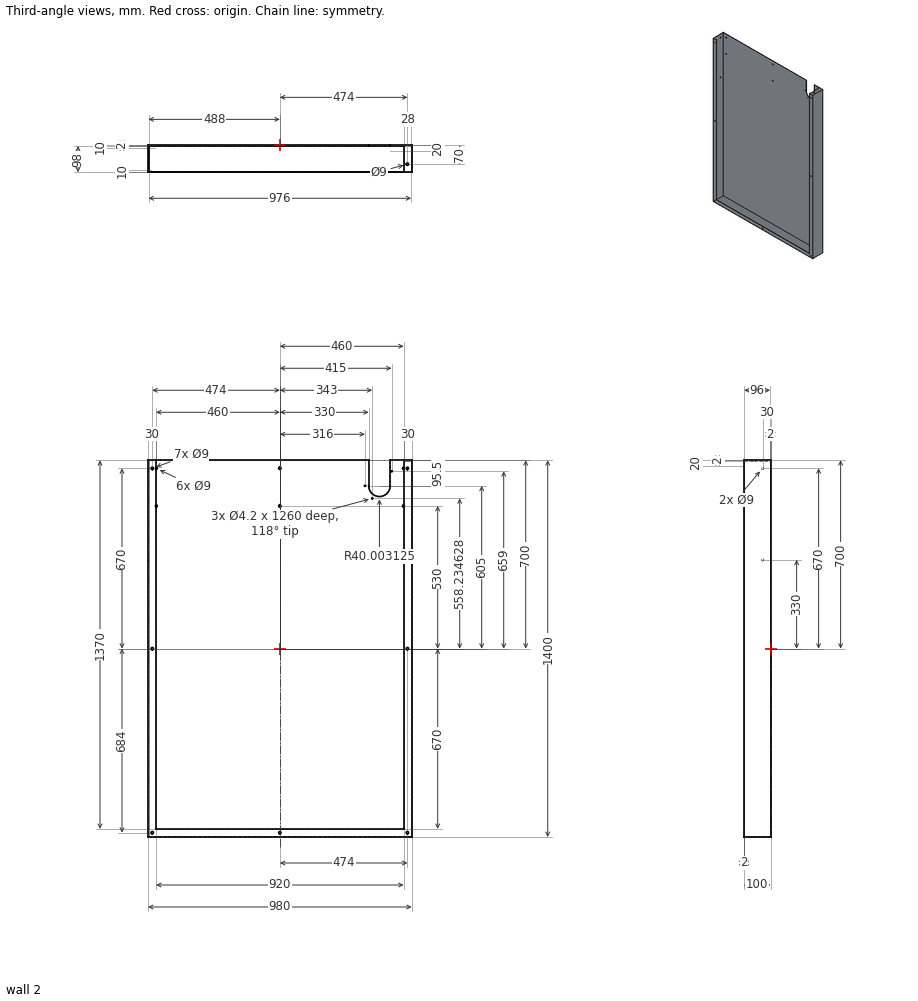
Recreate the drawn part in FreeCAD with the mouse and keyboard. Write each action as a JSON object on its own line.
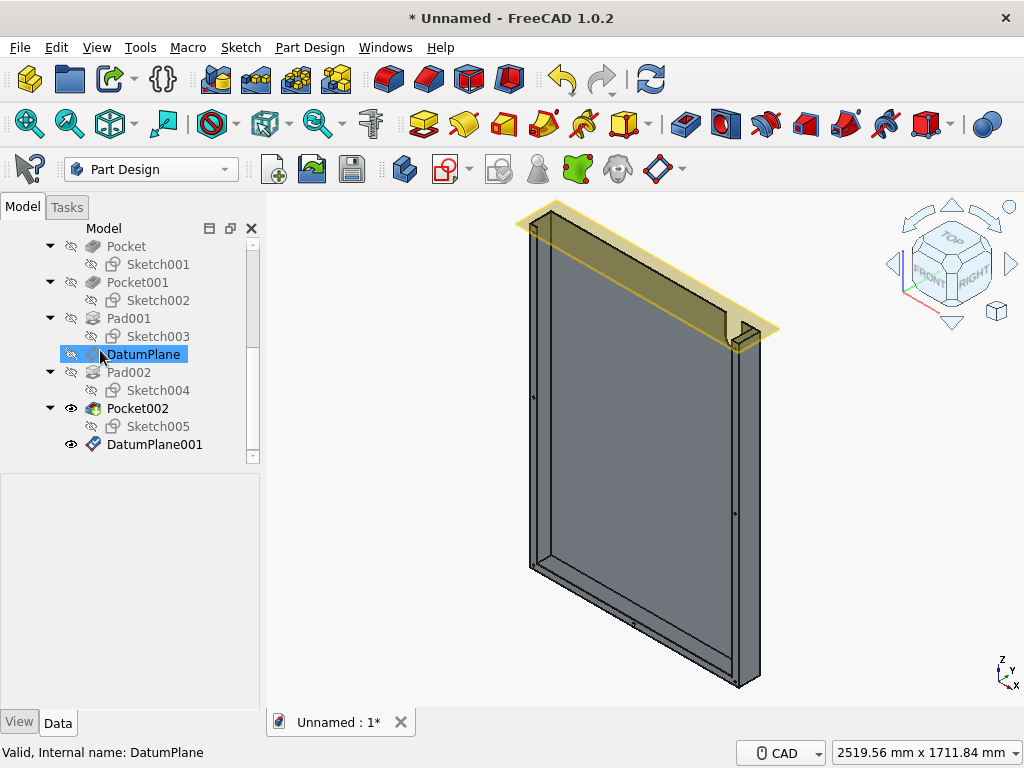
{"action": "left_click", "coordinate": [116, 444]}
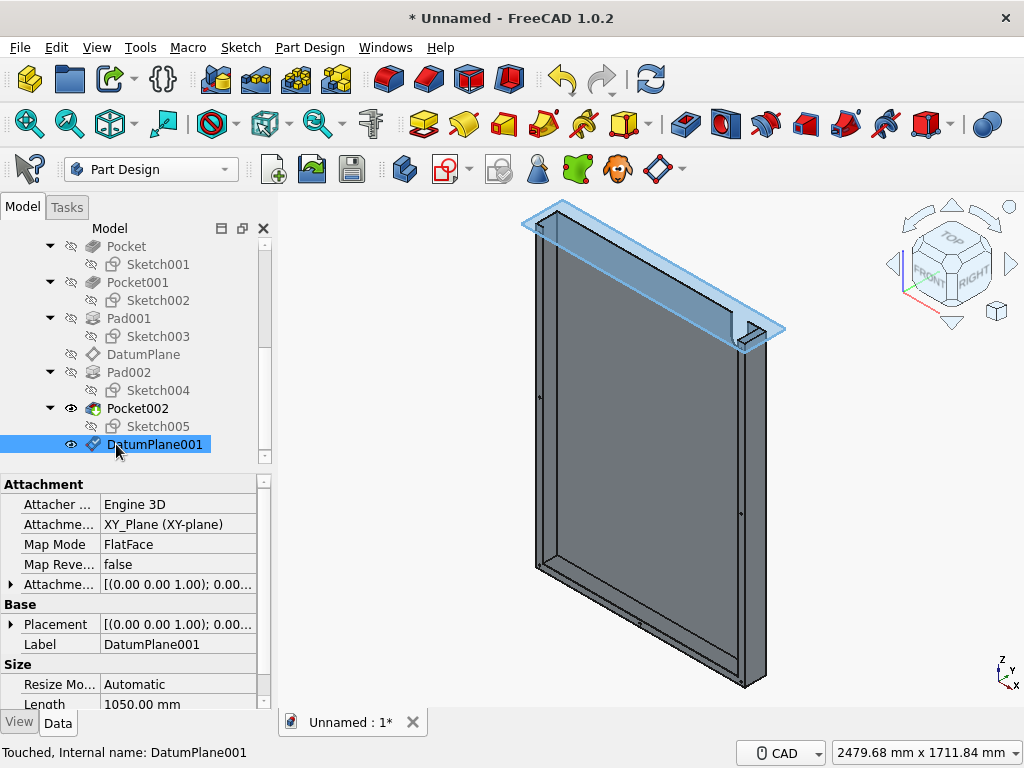
{"action": "left_click", "coordinate": [446, 170]}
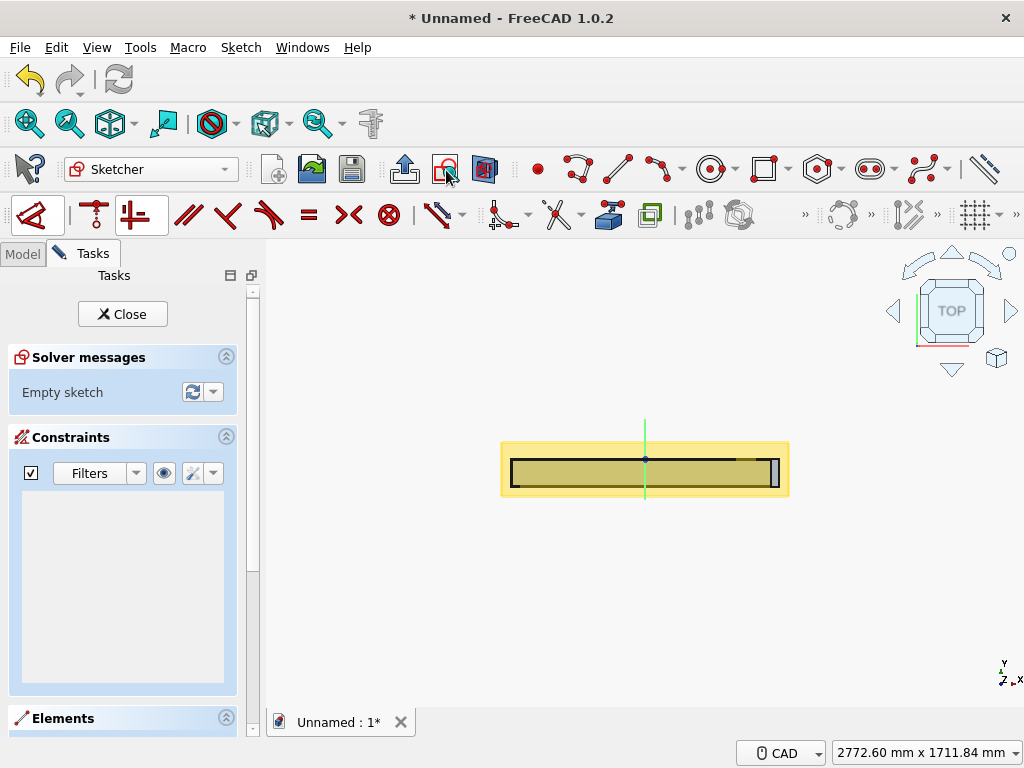
{"action": "left_click", "coordinate": [486, 170]}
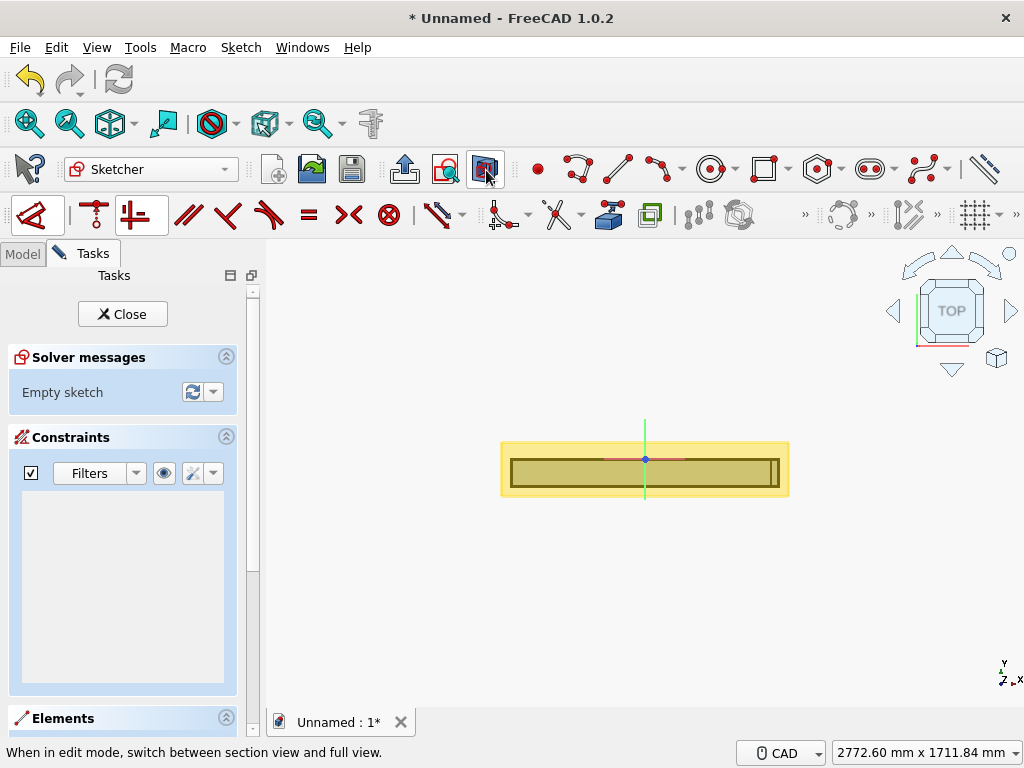
{"action": "scroll", "coordinate": [785, 479], "scroll_direction": "up", "scroll_amount": 15}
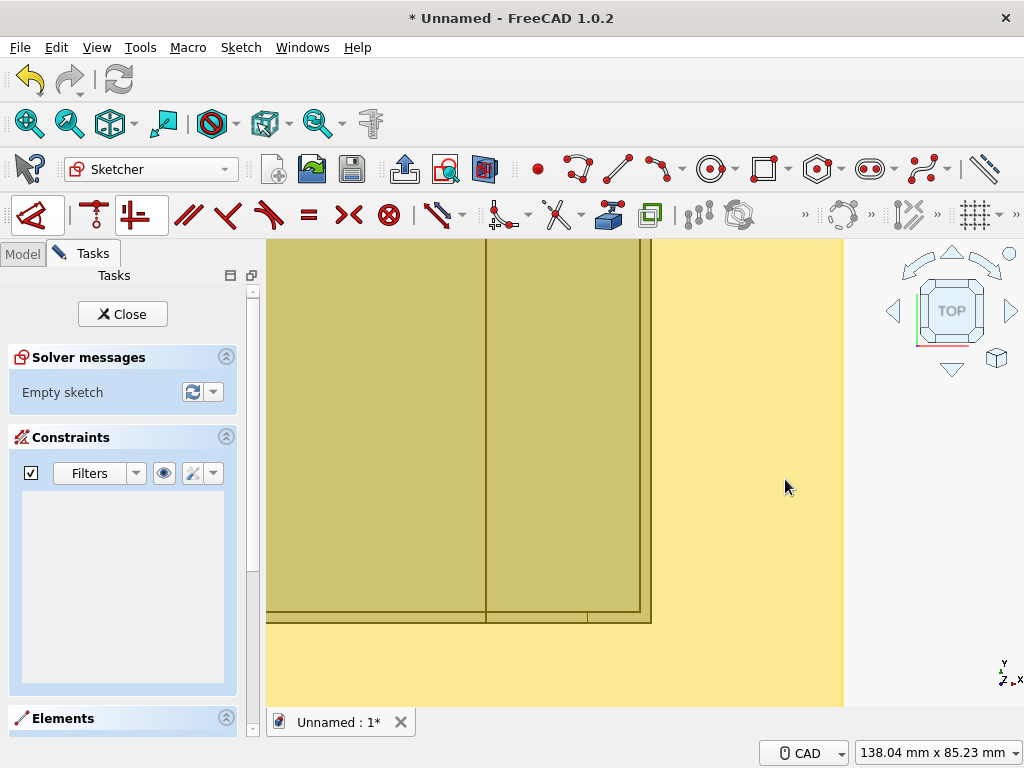
{"action": "scroll", "coordinate": [560, 456], "scroll_direction": "up", "scroll_amount": 9}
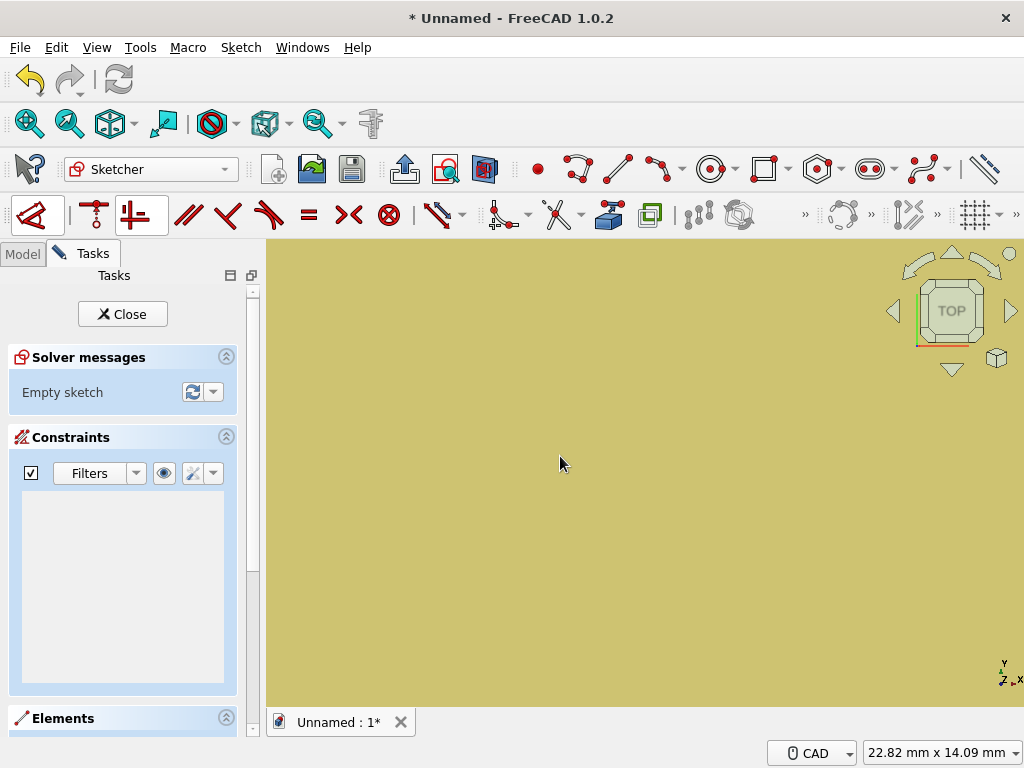
{"action": "left_click", "coordinate": [712, 170]}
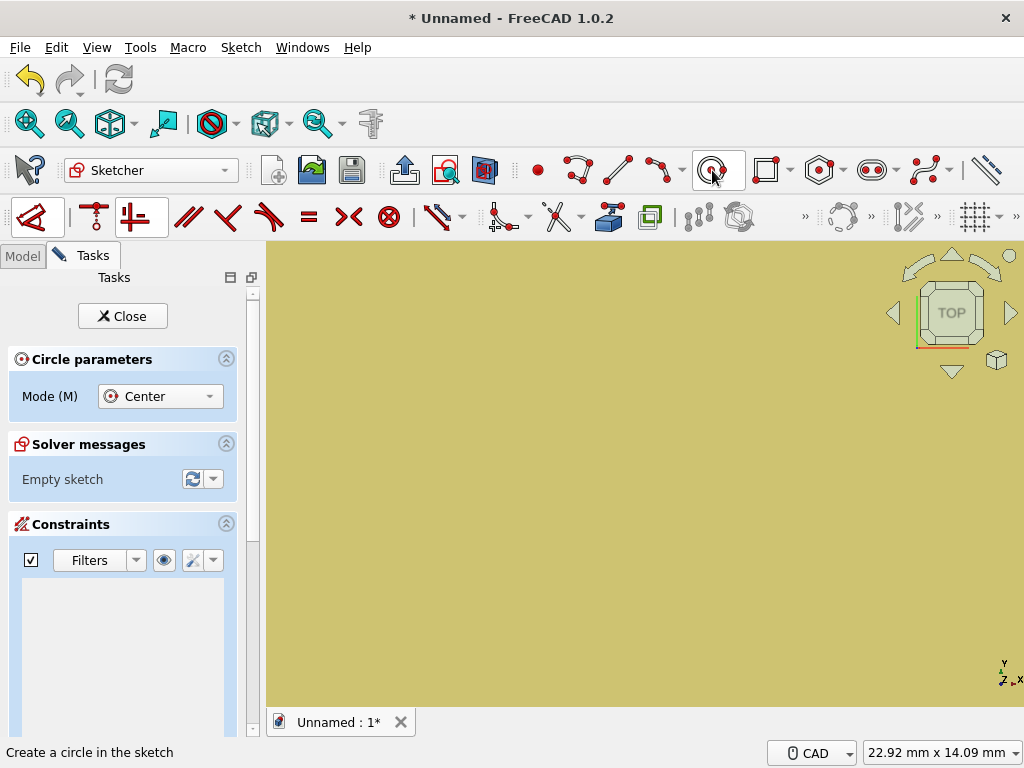
{"action": "left_click", "coordinate": [575, 470]}
{"action": "mouse_move", "coordinate": [680, 365]}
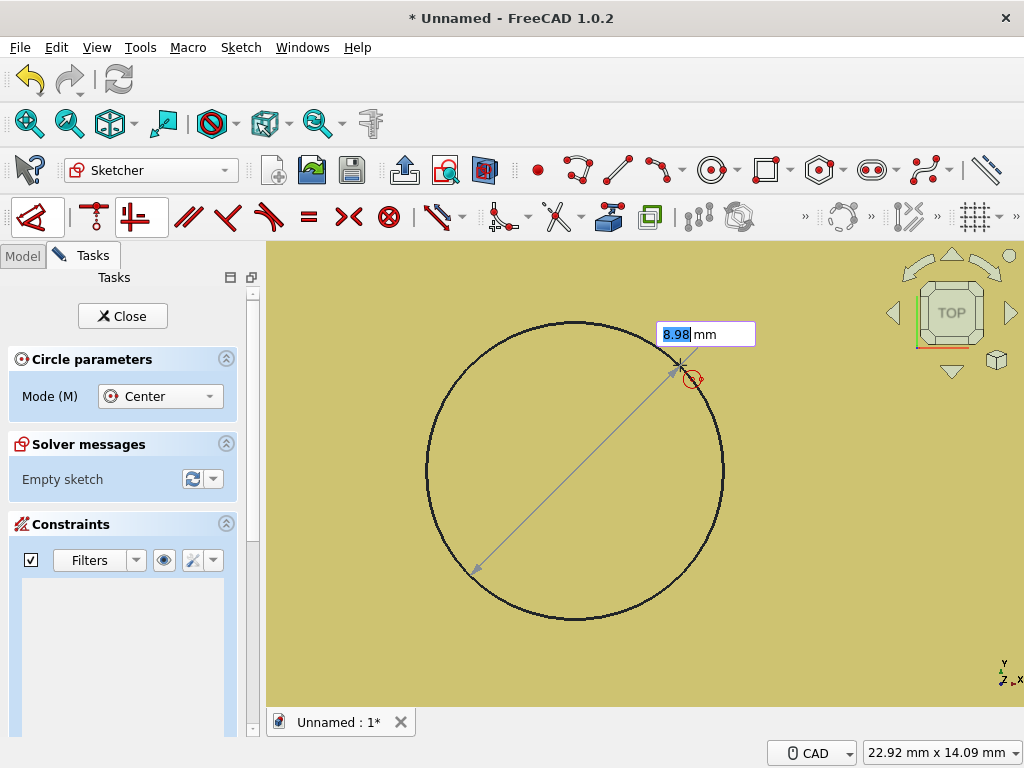
{"action": "type", "text": "9"}
{"action": "key", "text": "Return"}
{"action": "key", "text": "Escape"}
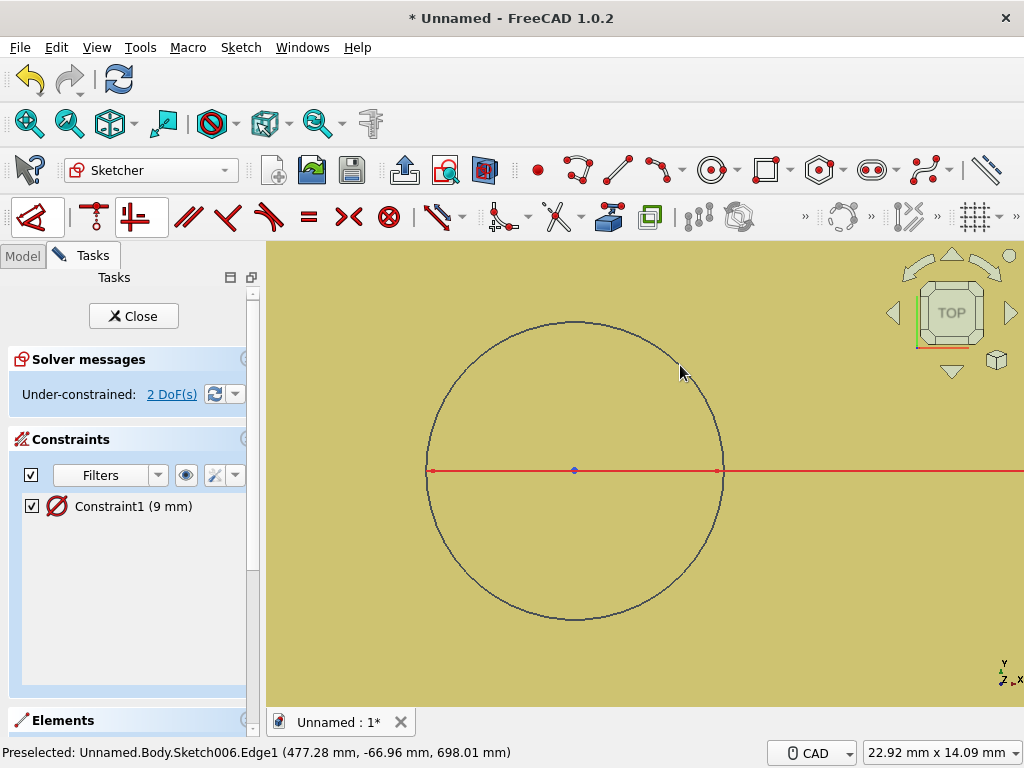
{"action": "left_click", "coordinate": [575, 471]}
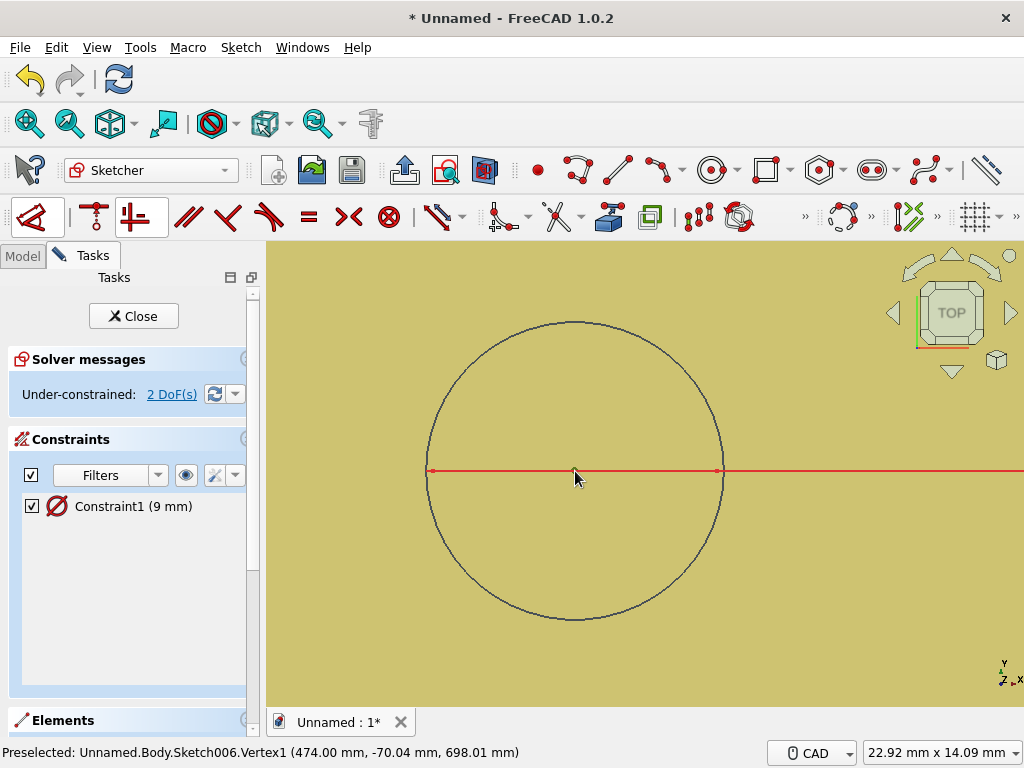
{"action": "left_click", "coordinate": [58, 218]}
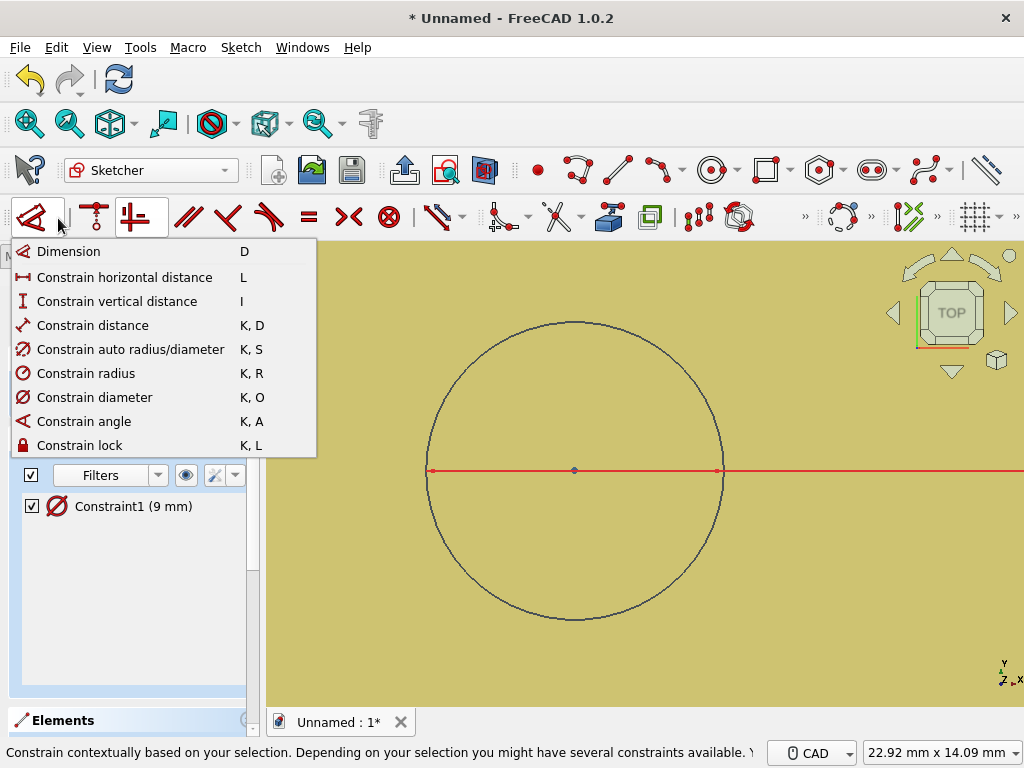
{"action": "left_click", "coordinate": [164, 301]}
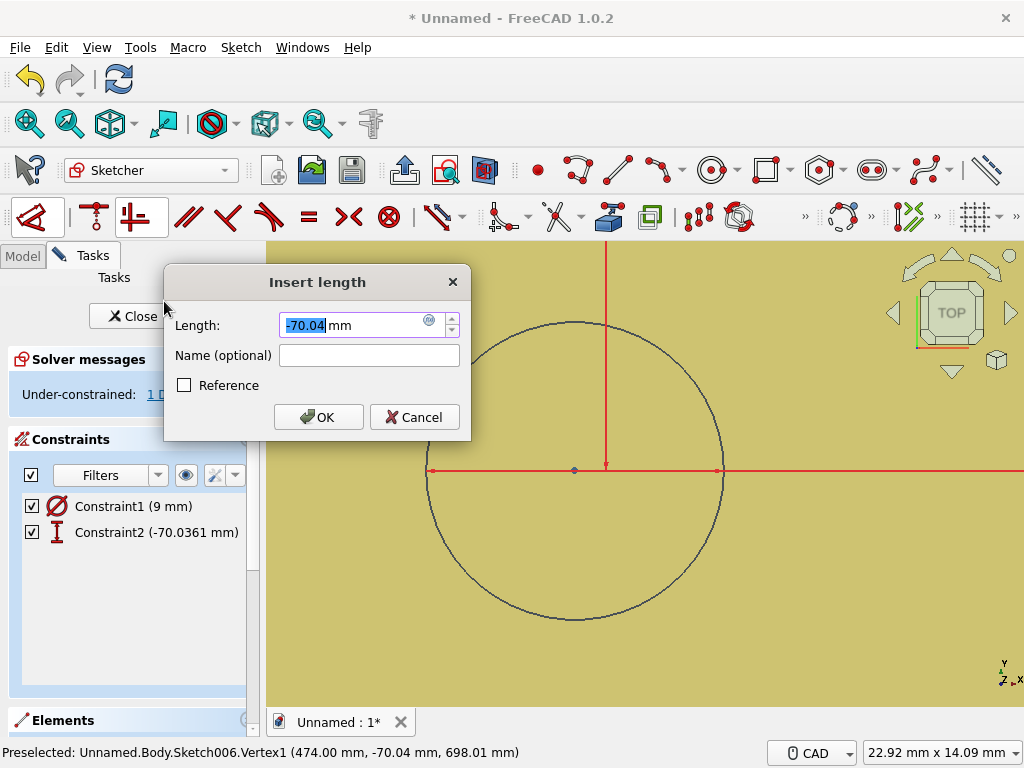
{"action": "type", "text": "-70"}
{"action": "key", "text": "Return"}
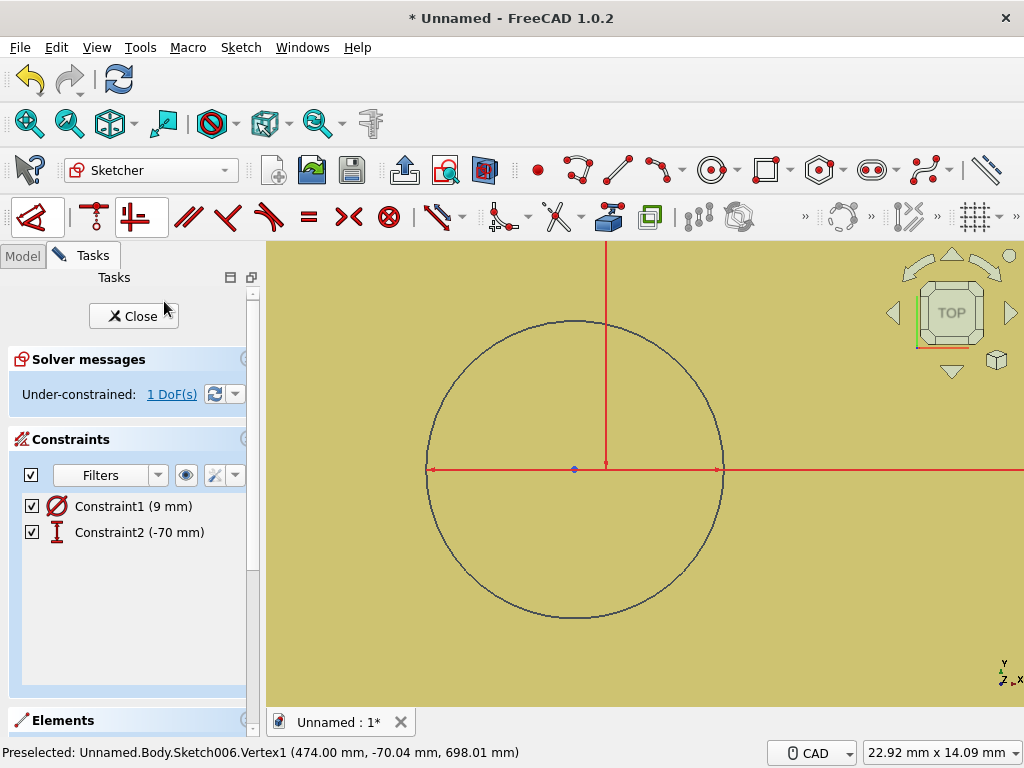
{"action": "left_click", "coordinate": [575, 470]}